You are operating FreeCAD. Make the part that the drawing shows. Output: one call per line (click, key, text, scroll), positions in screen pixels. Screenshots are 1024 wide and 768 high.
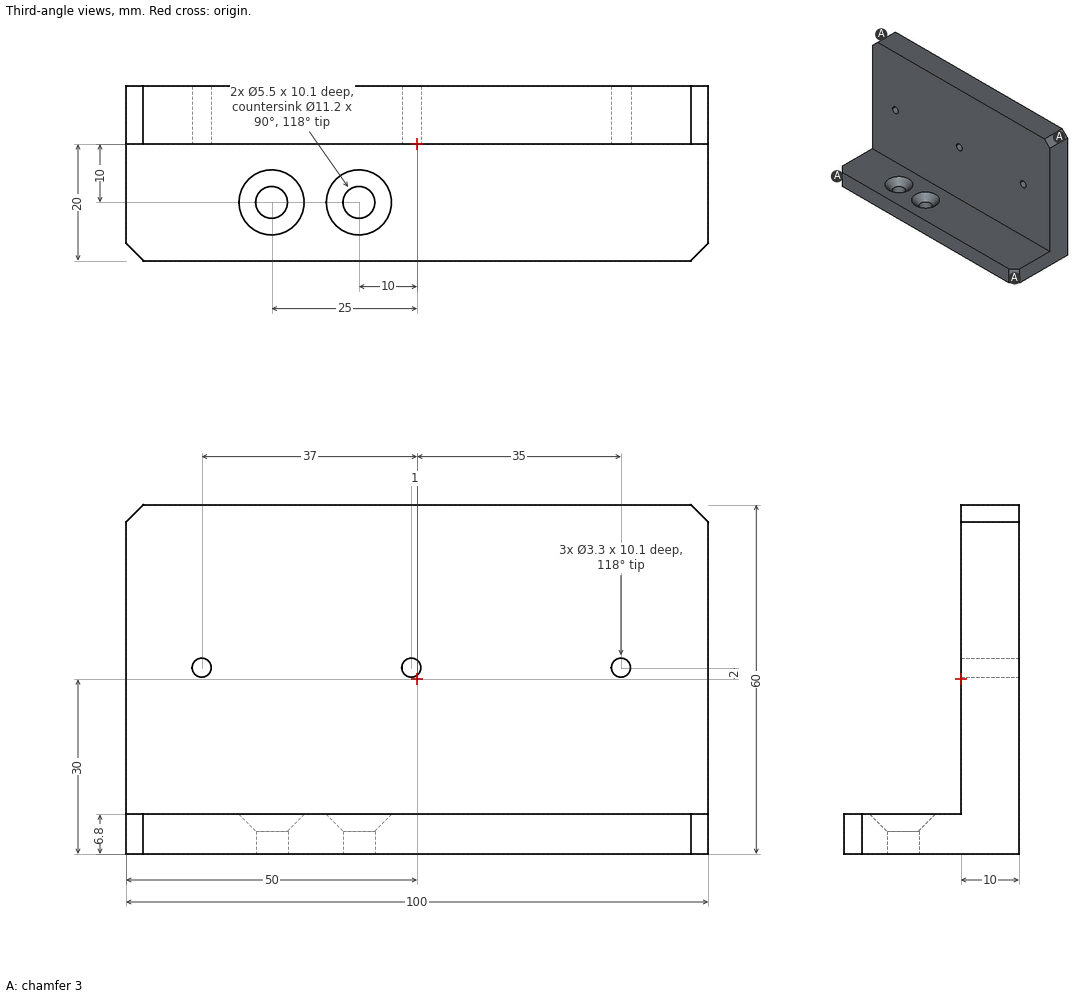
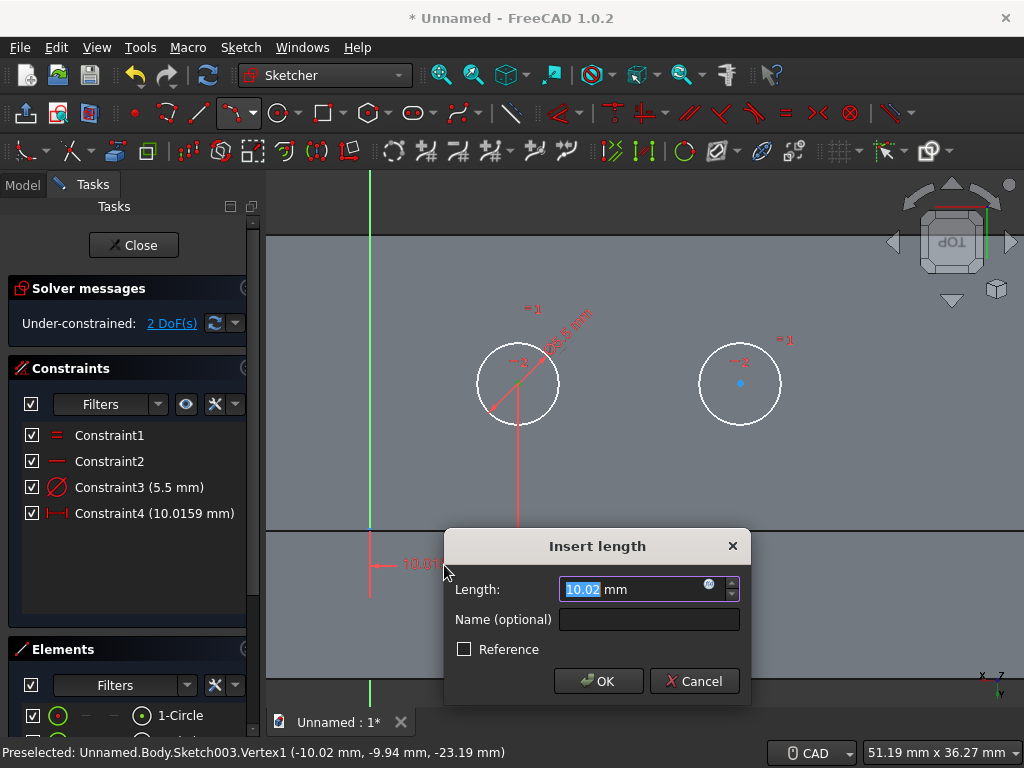
text(10)
key(Return)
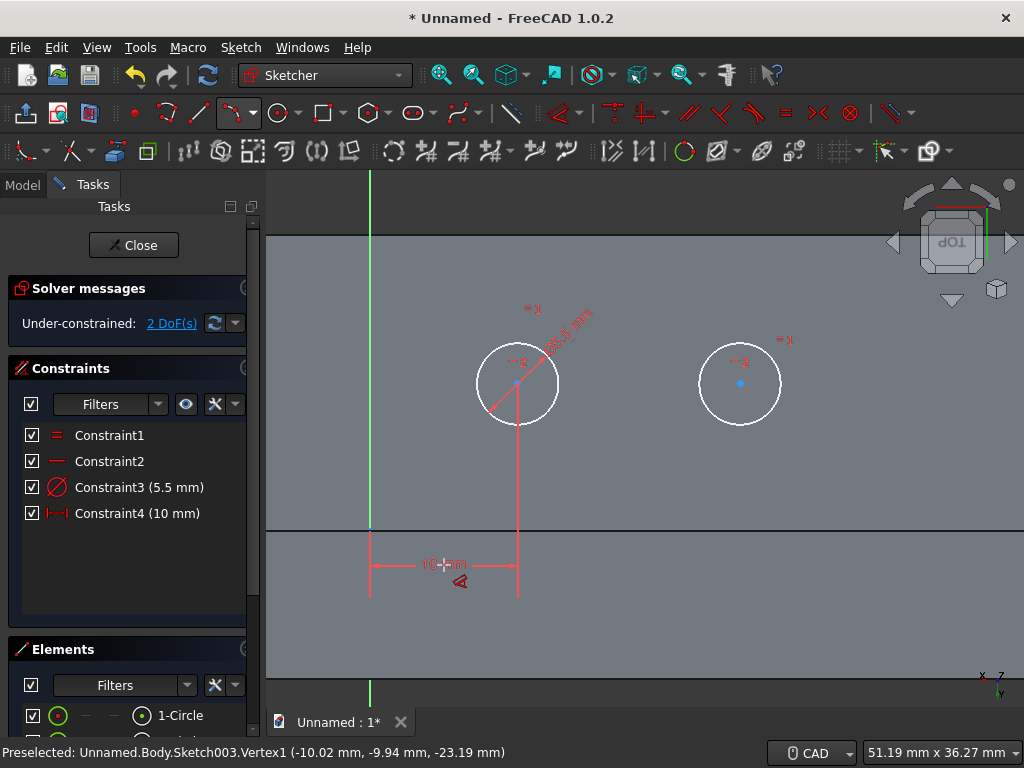
click(518, 384)
click(336, 458)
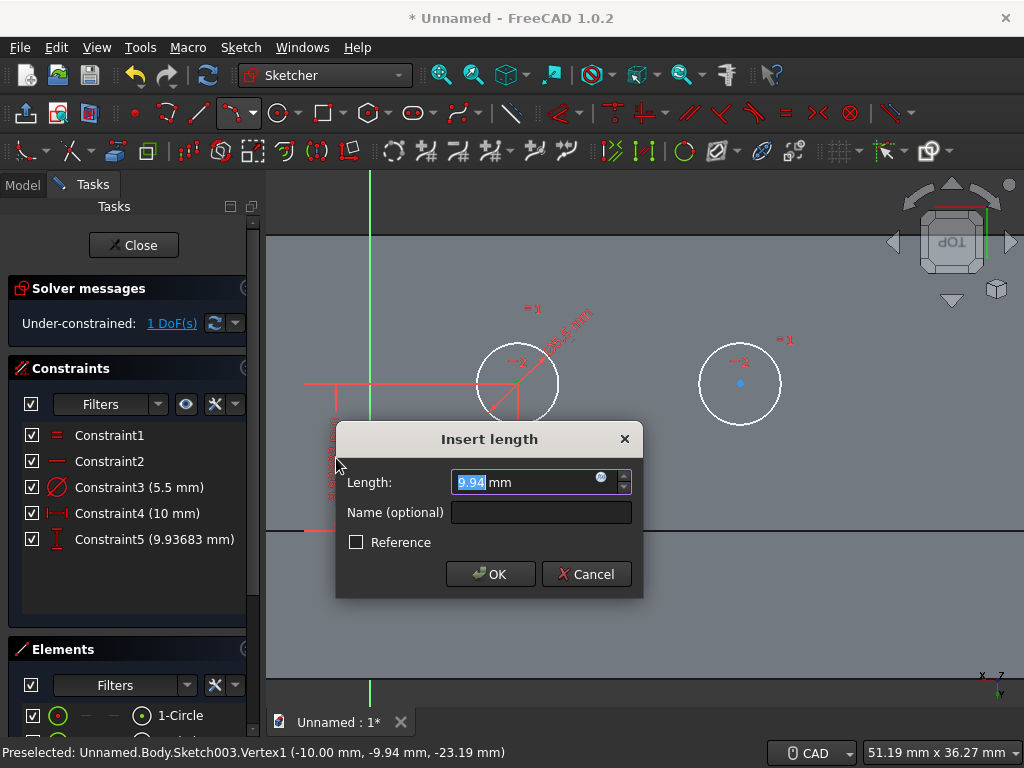
text(10)
key(Return)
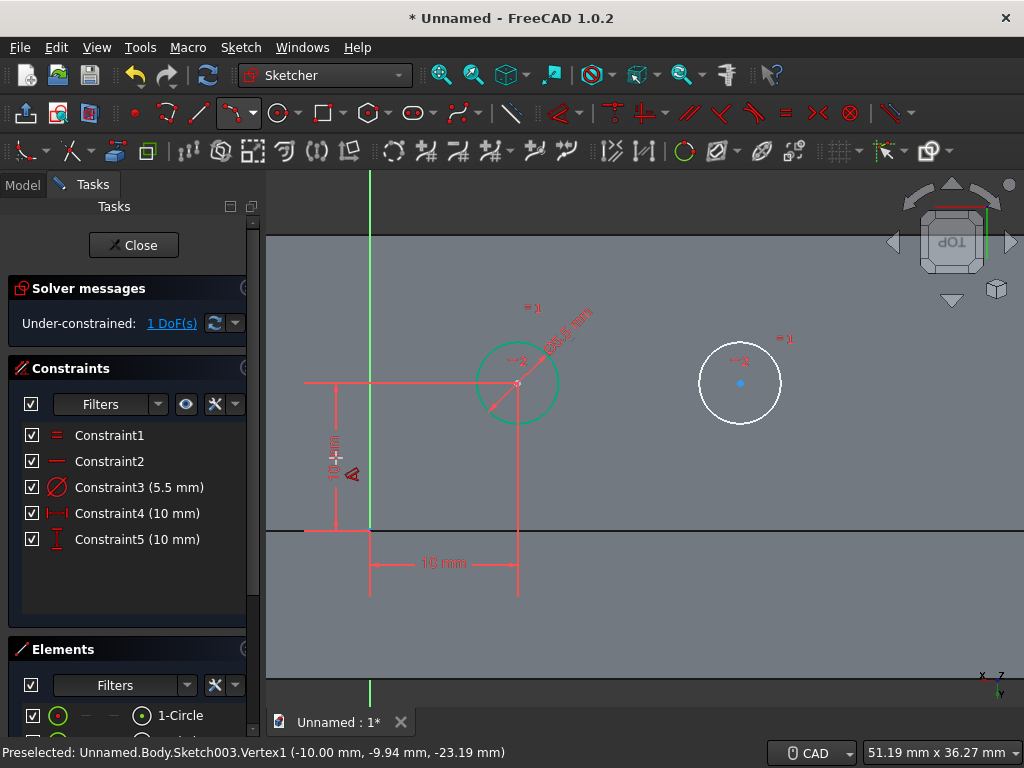
click(740, 383)
click(555, 565)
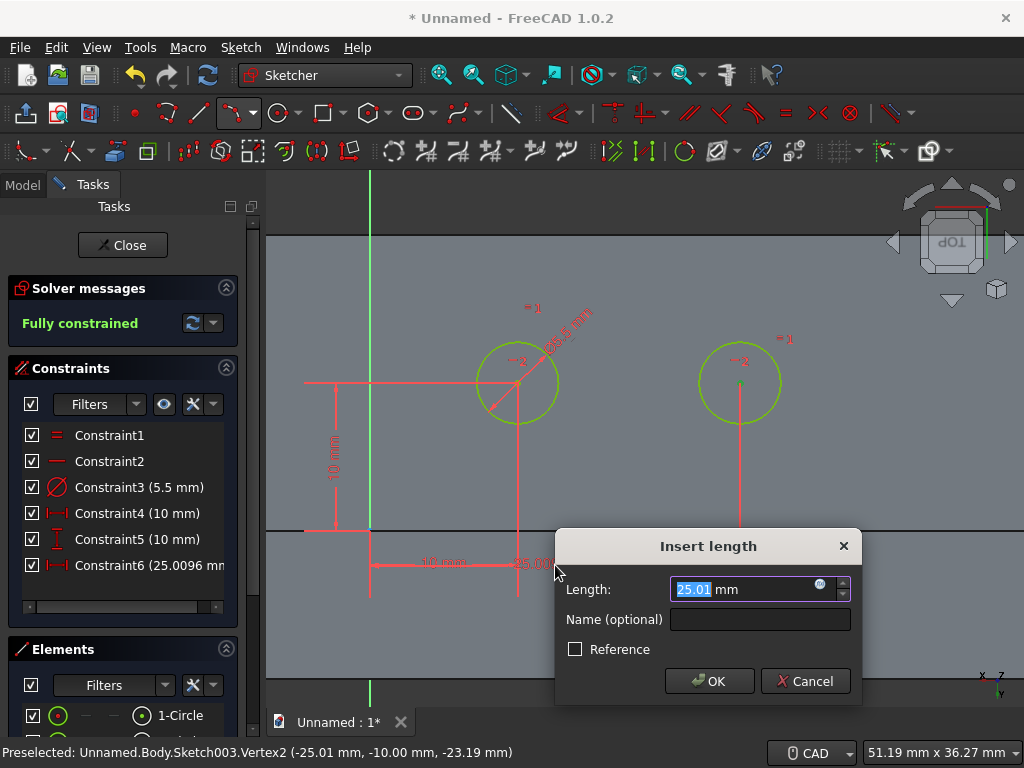
text(25)
key(Return)
key(Escape)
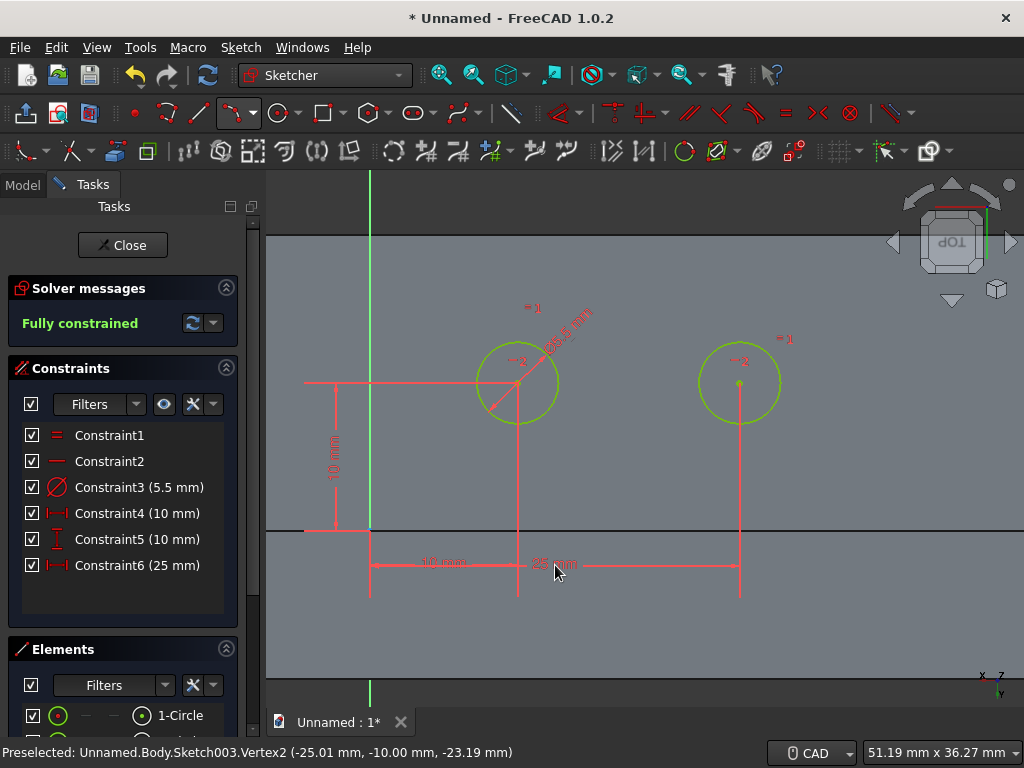
click(123, 245)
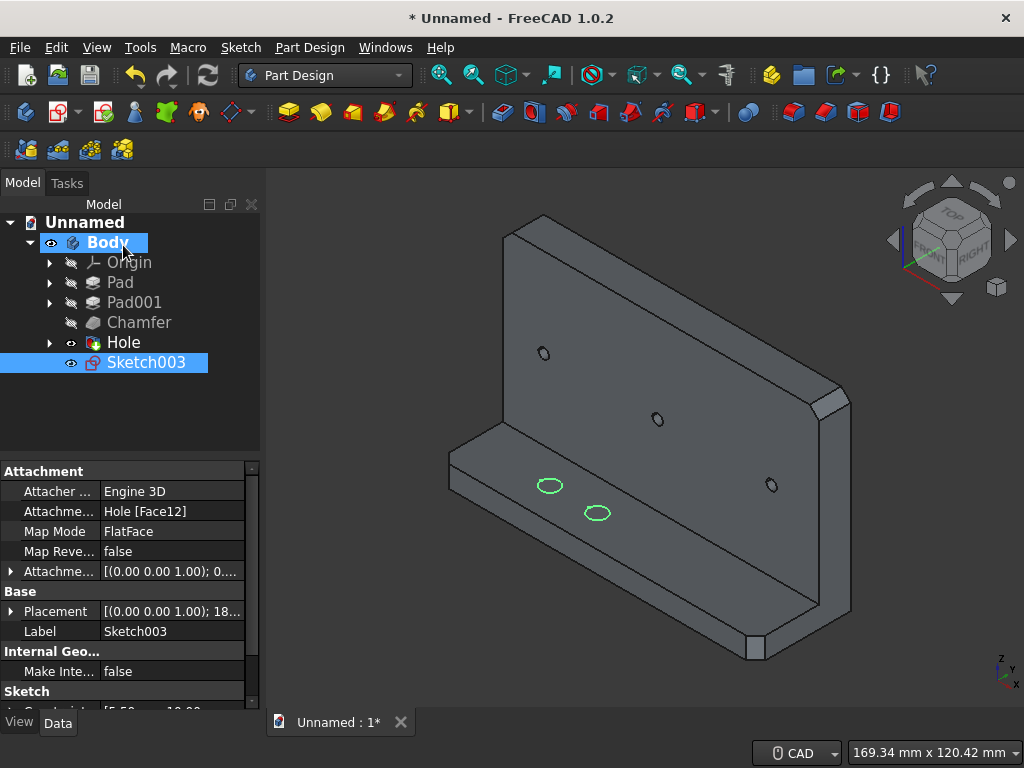
click(536, 112)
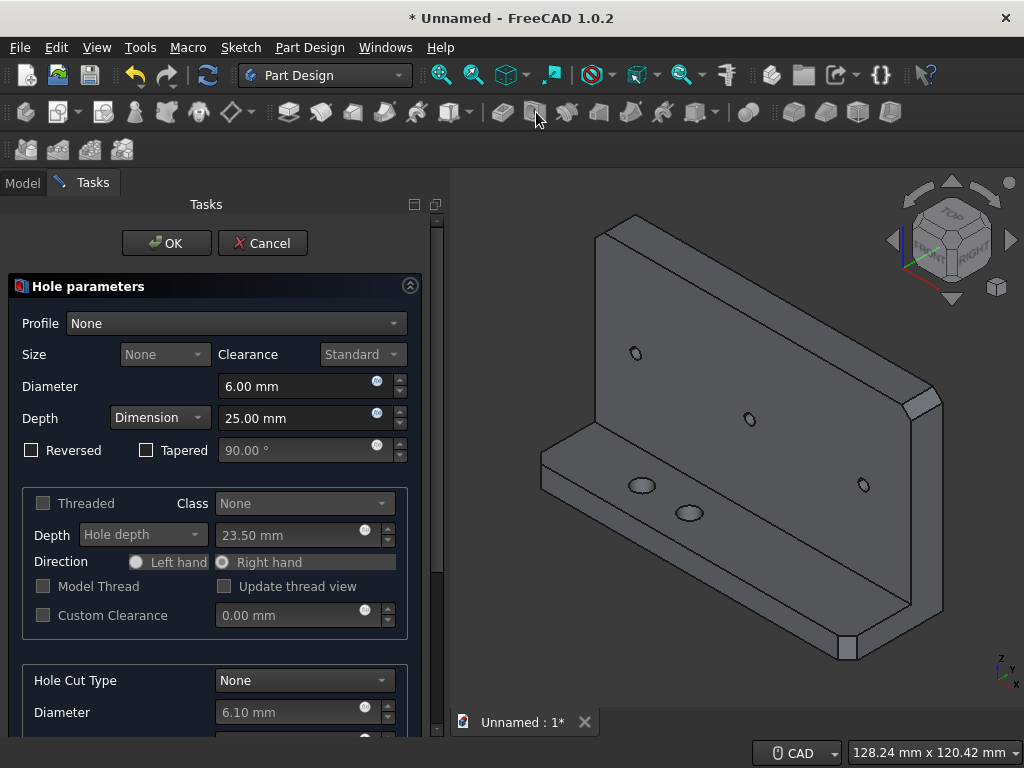
triple_click(305, 386)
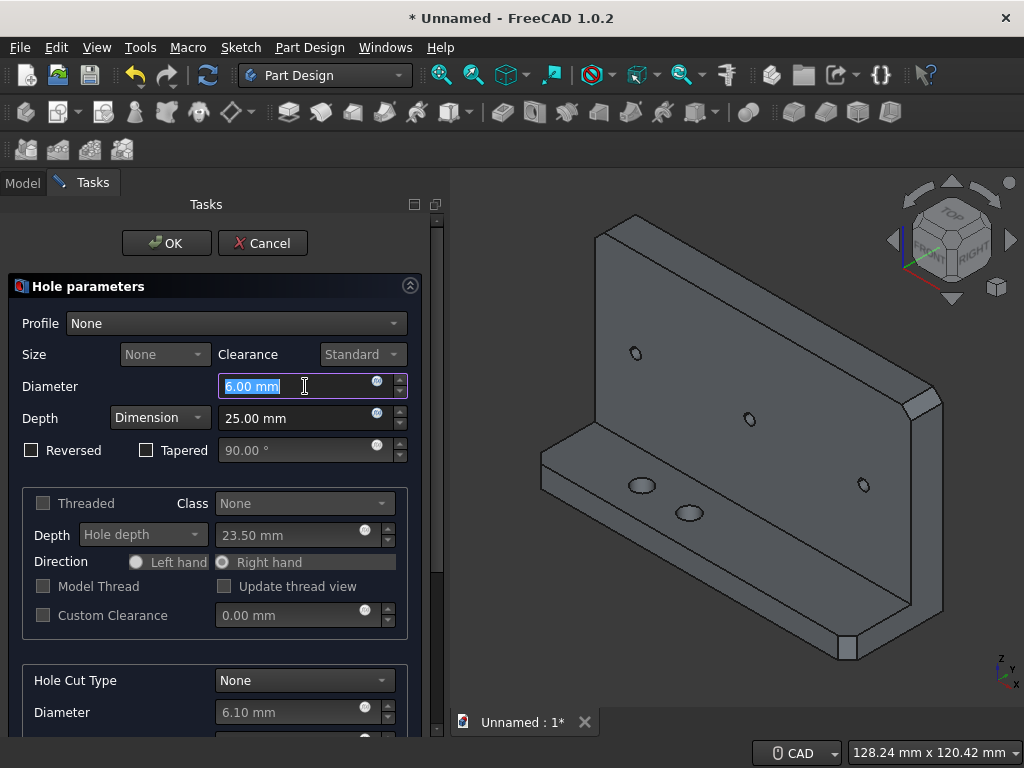
text(5.5)
key(Tab)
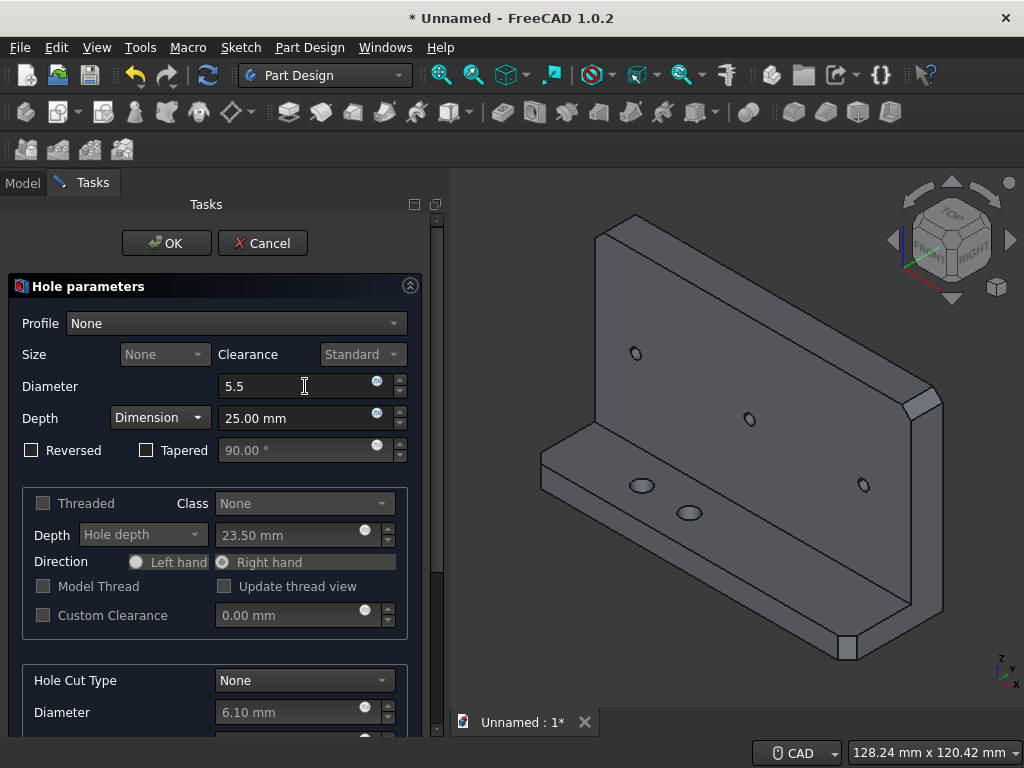
triple_click(305, 418)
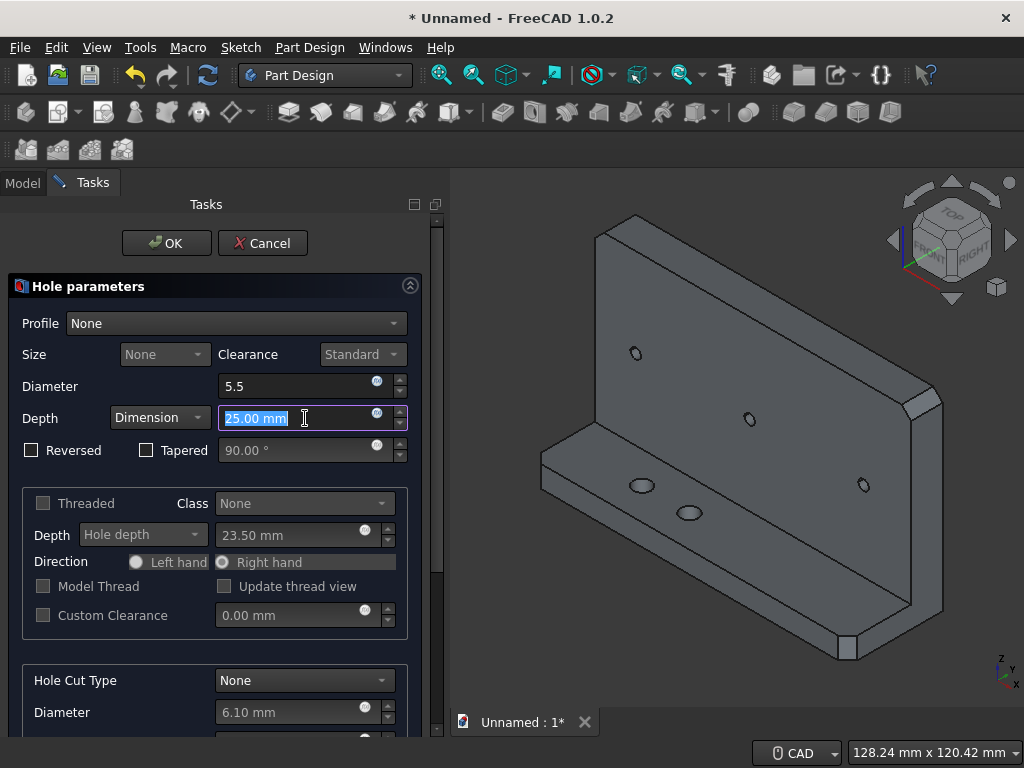
text(10.1)
key(Tab)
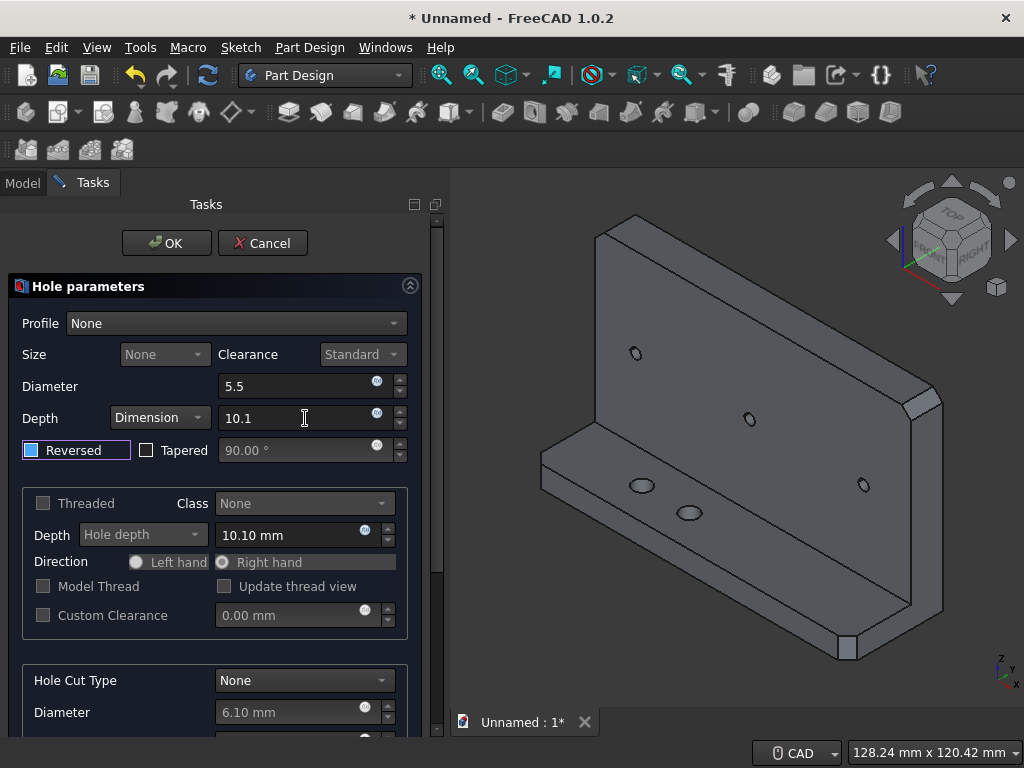
click(306, 680)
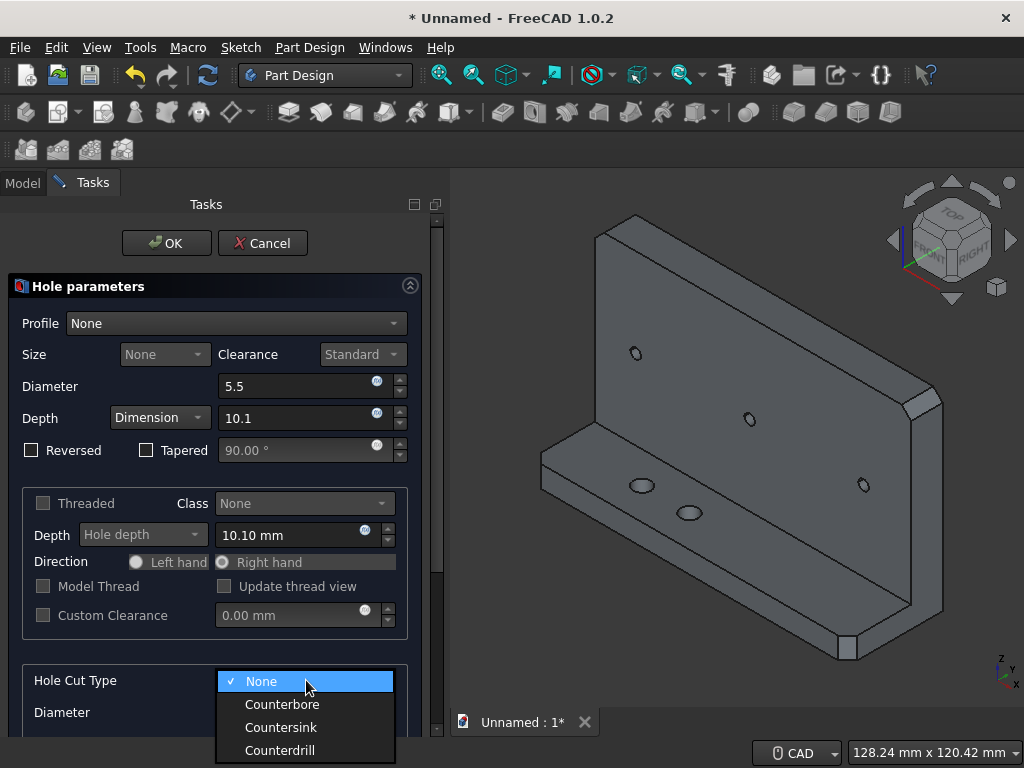
click(304, 728)